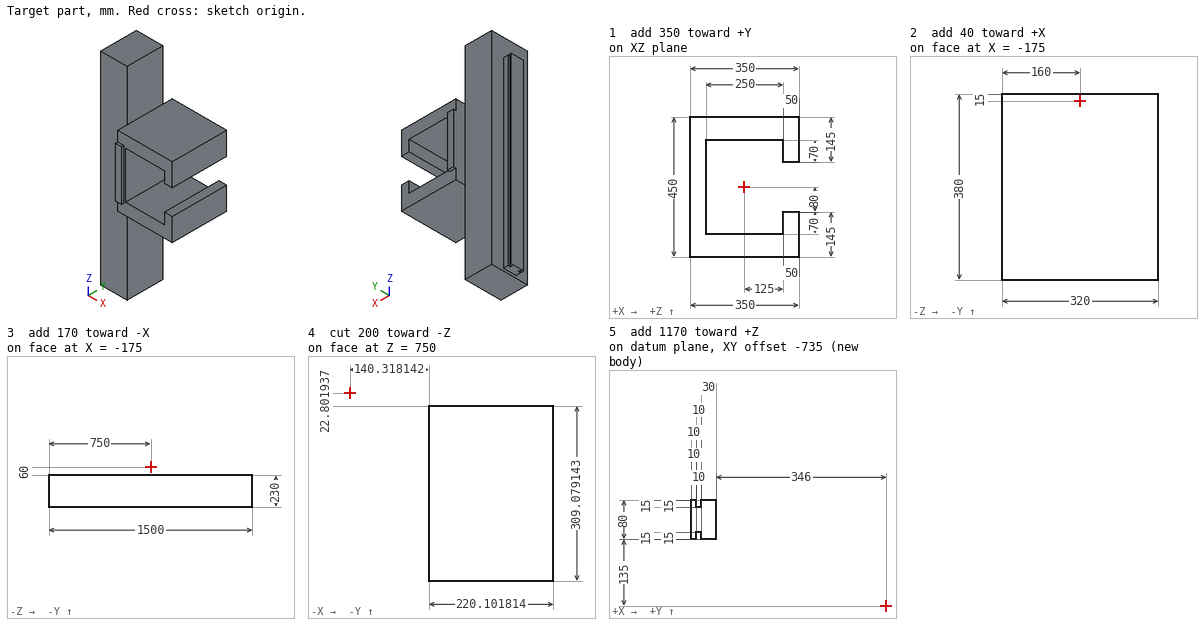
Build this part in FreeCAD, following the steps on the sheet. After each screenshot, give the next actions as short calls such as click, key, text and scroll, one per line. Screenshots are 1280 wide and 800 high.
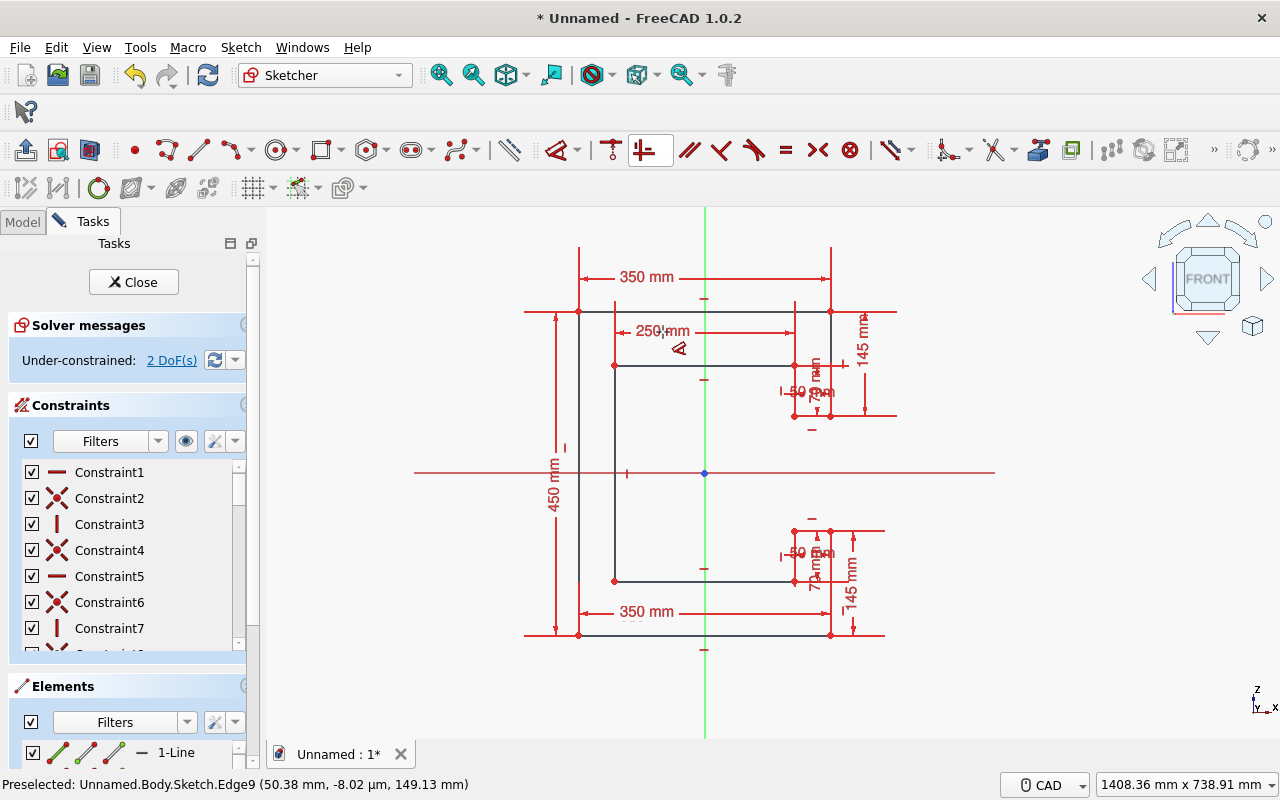
click(795, 531)
click(829, 502)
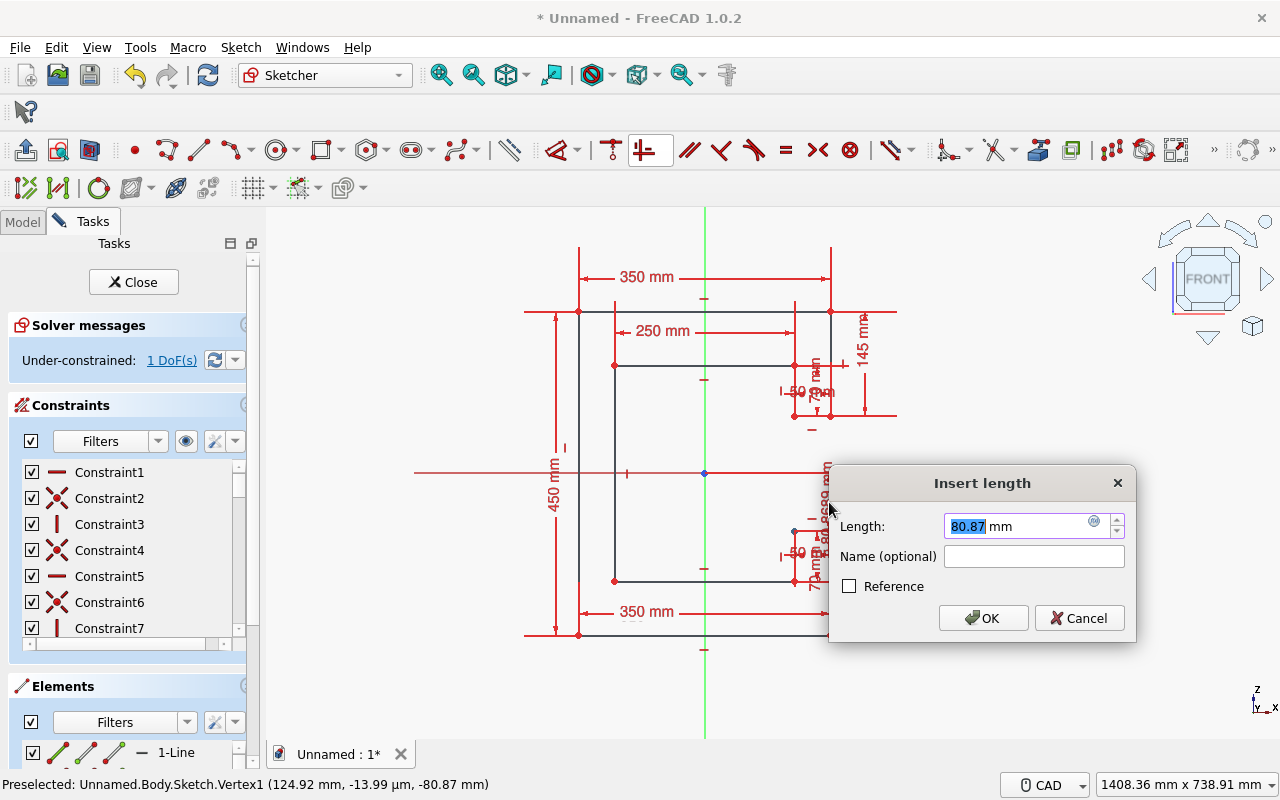
text(80)
key(Return)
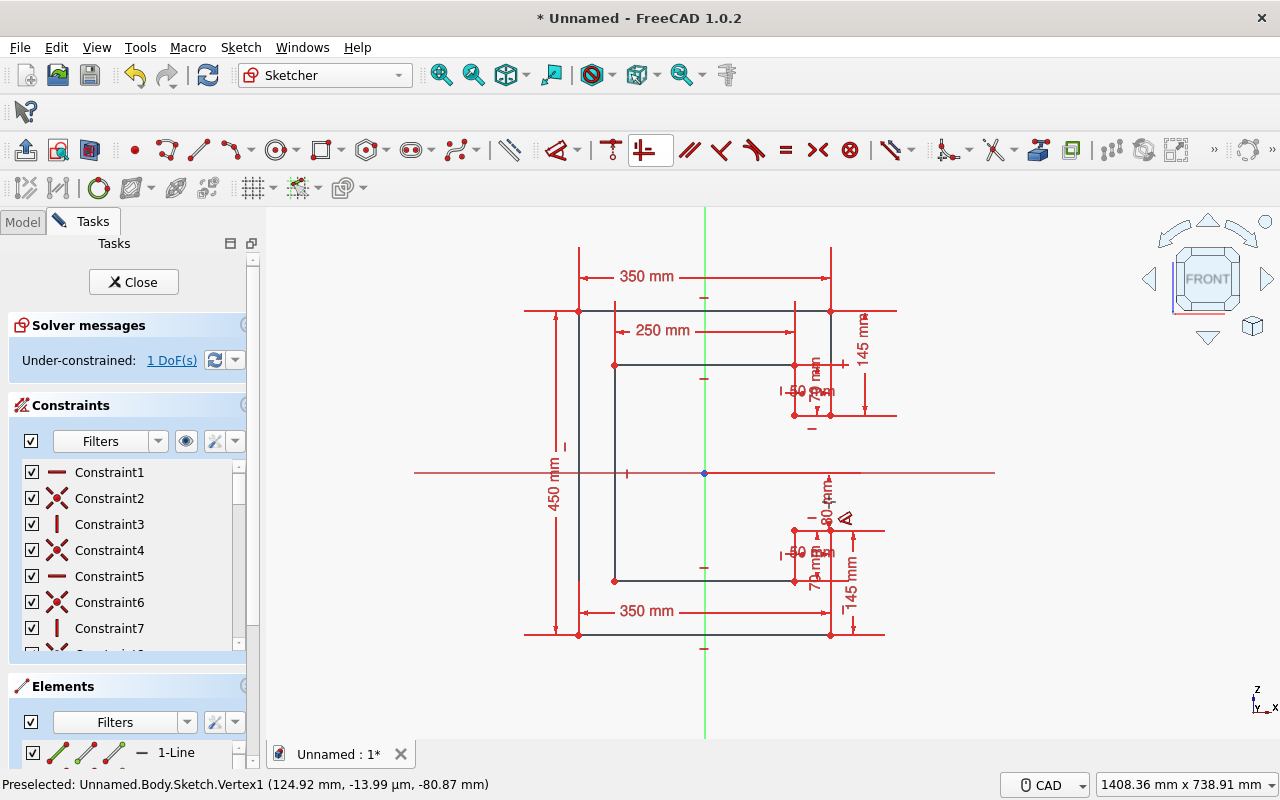
click(795, 531)
click(729, 565)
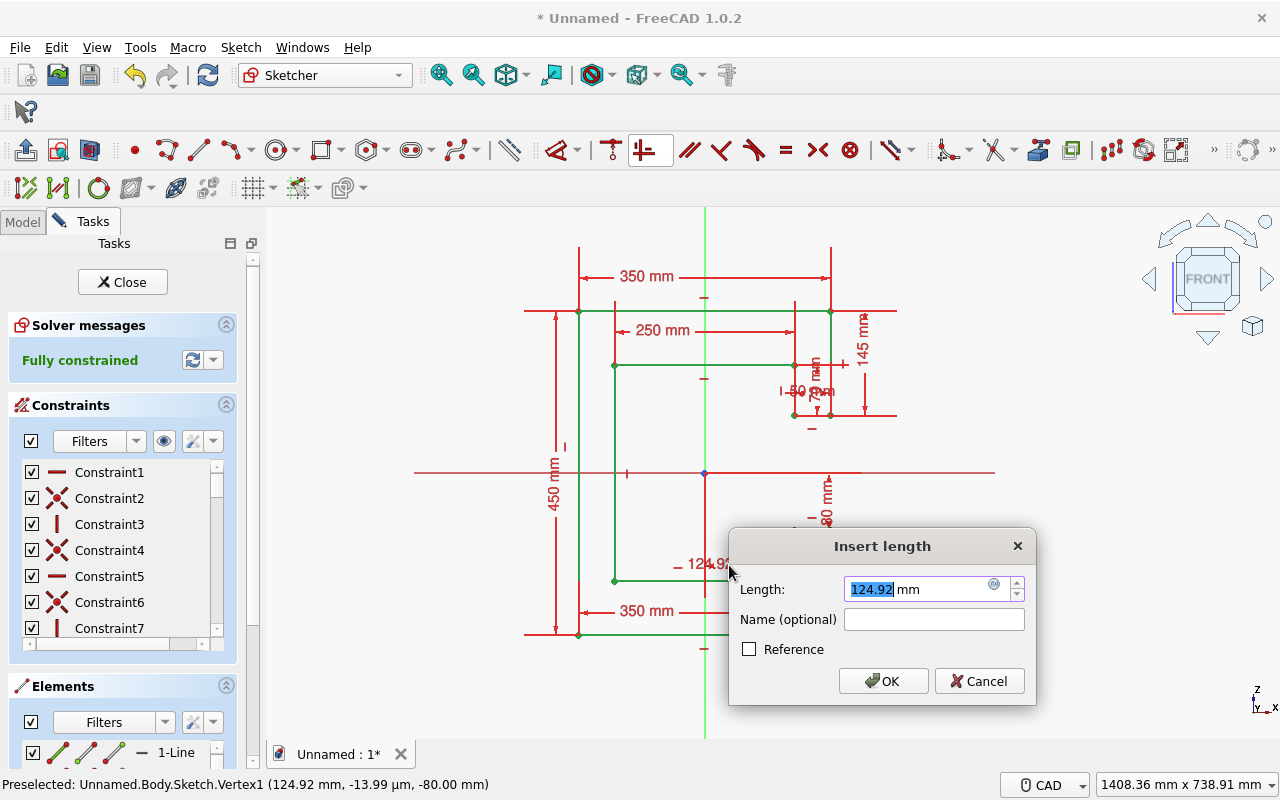
text(125)
key(Return)
key(Escape)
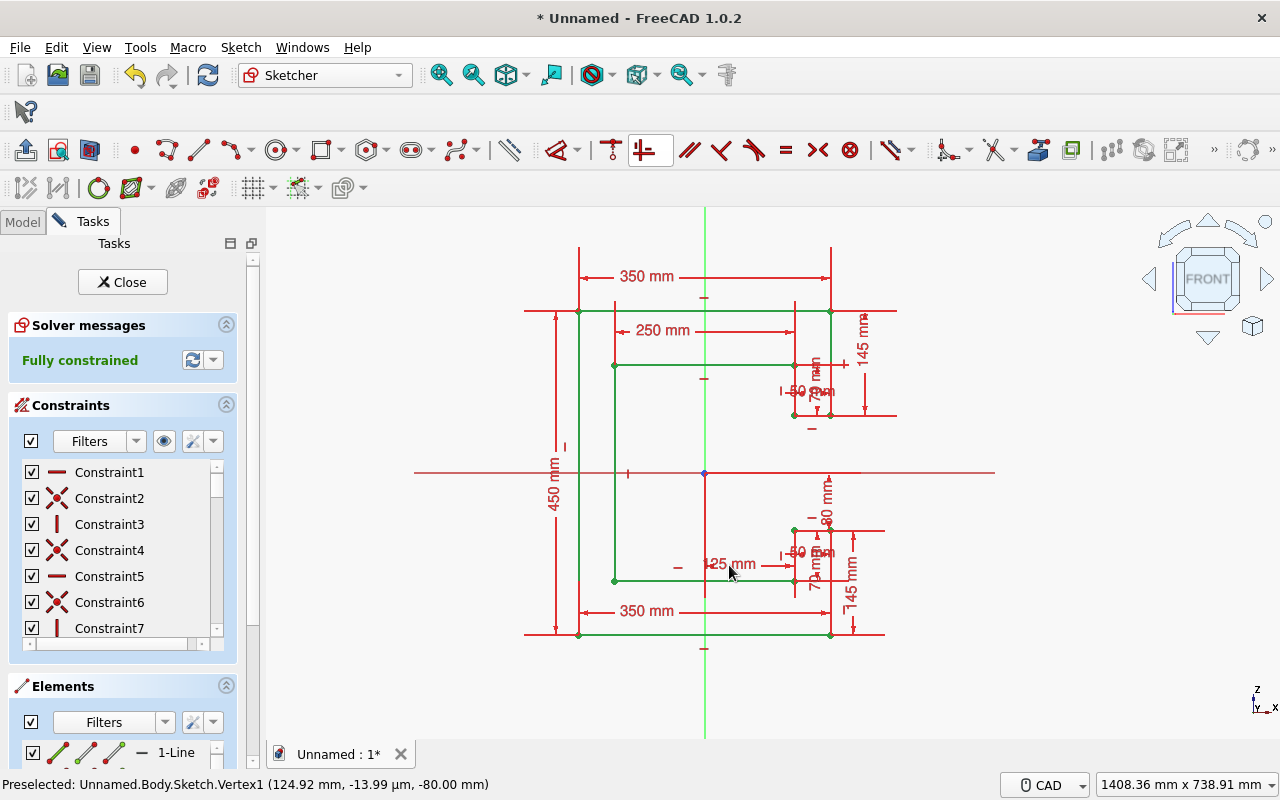
click(123, 282)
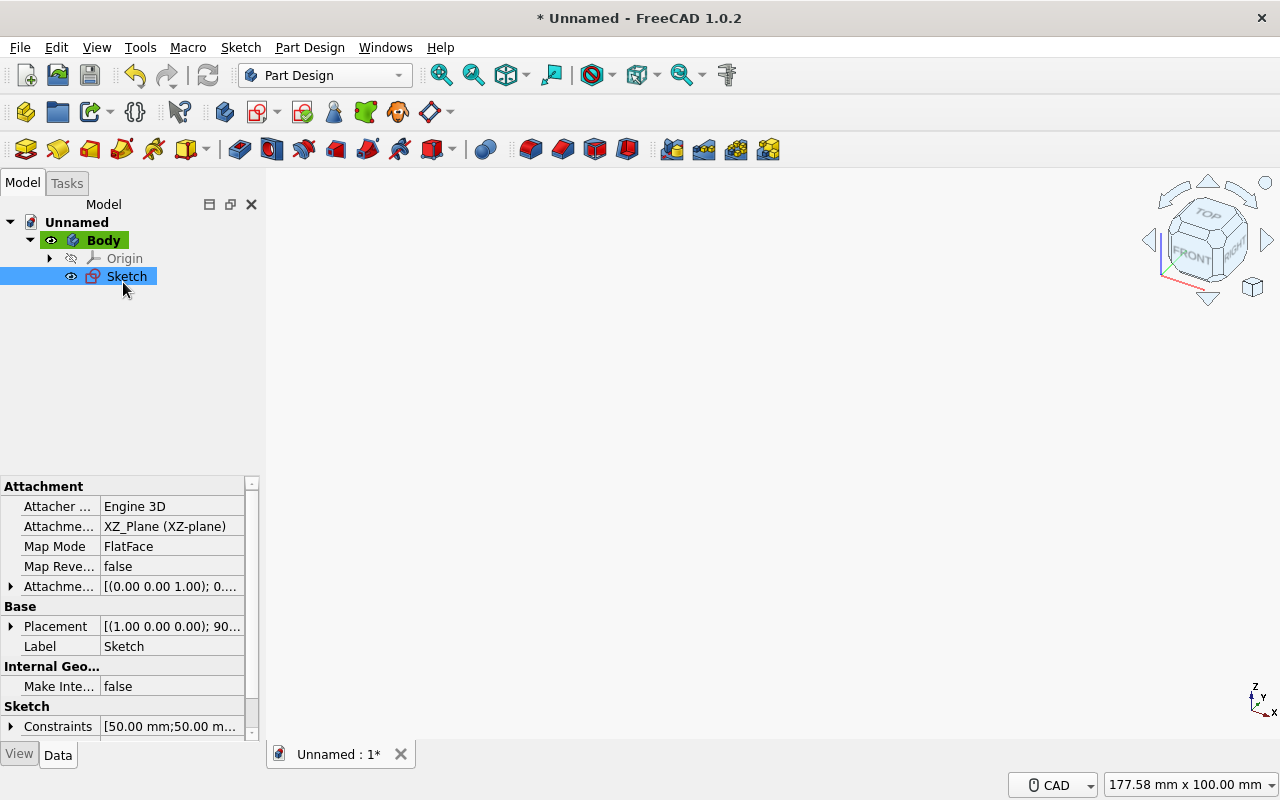
click(26, 150)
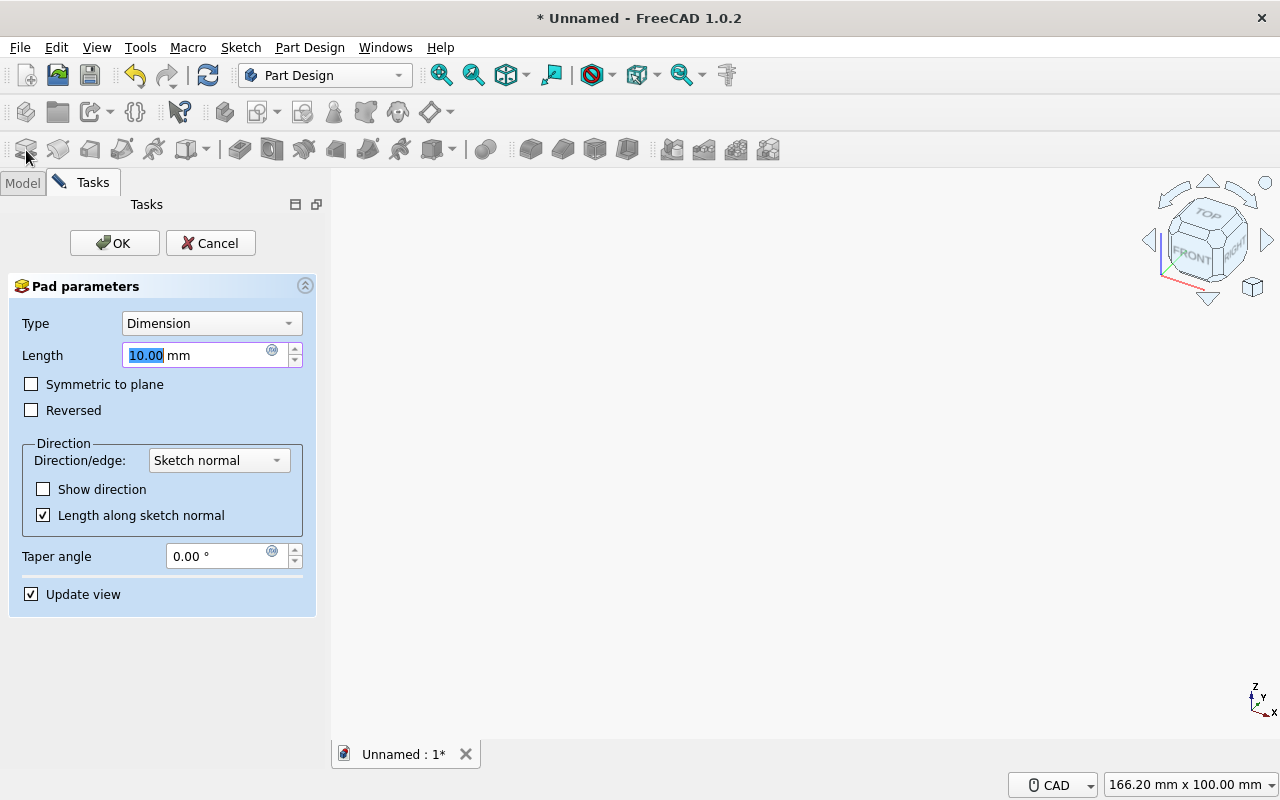
text(350)
key(Tab)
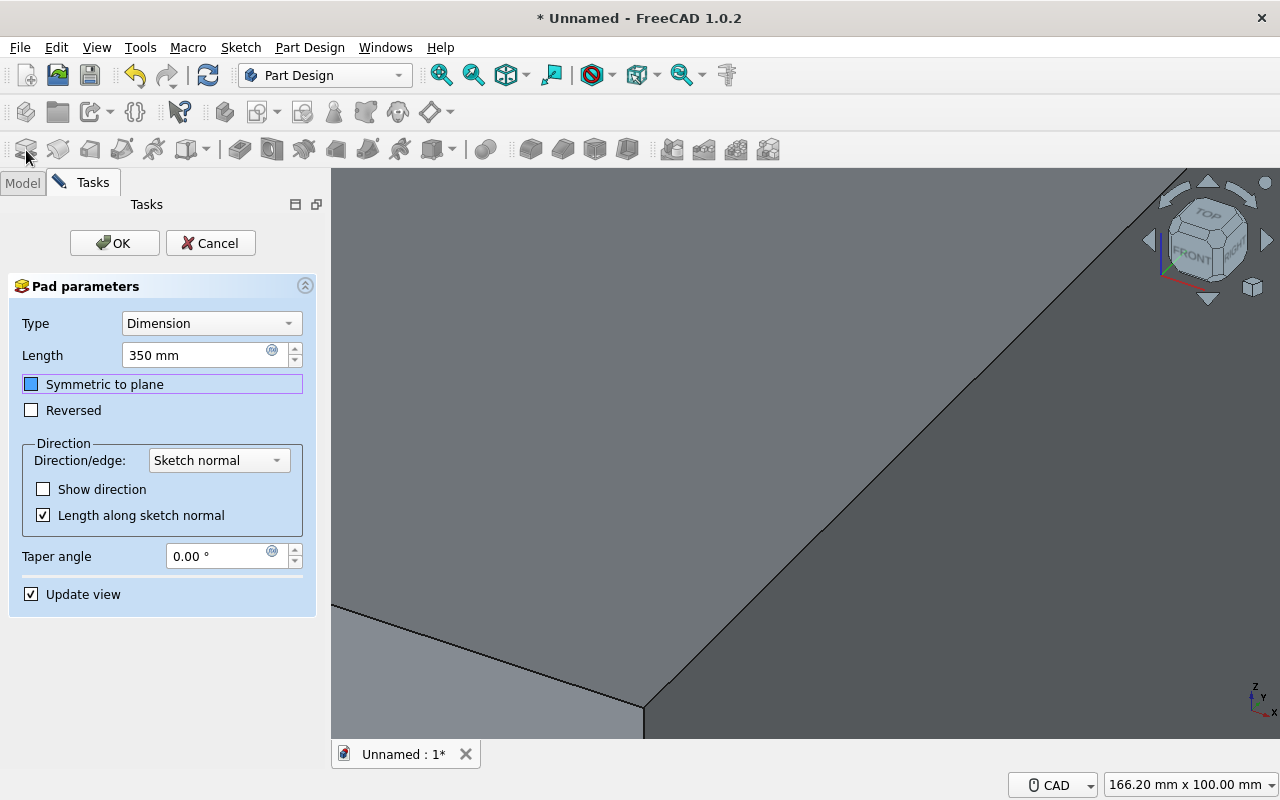
click(30, 410)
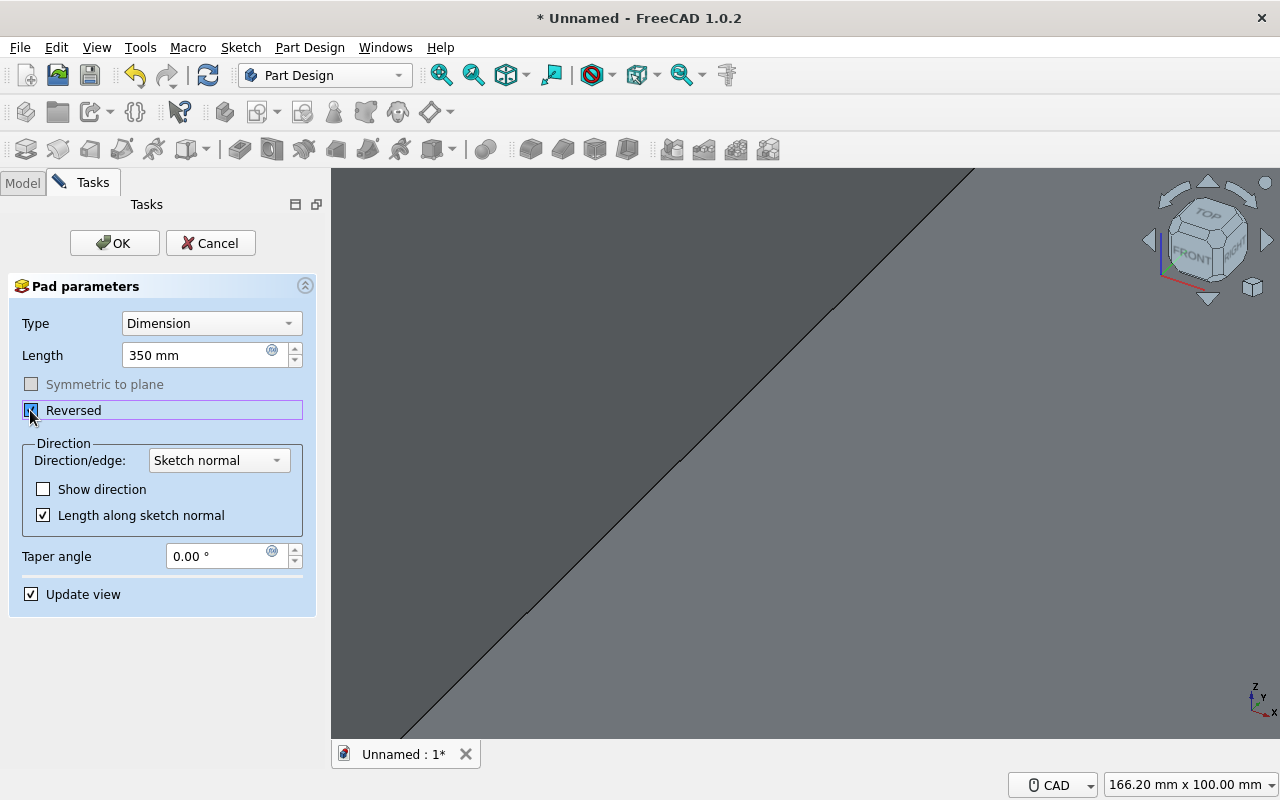
click(115, 243)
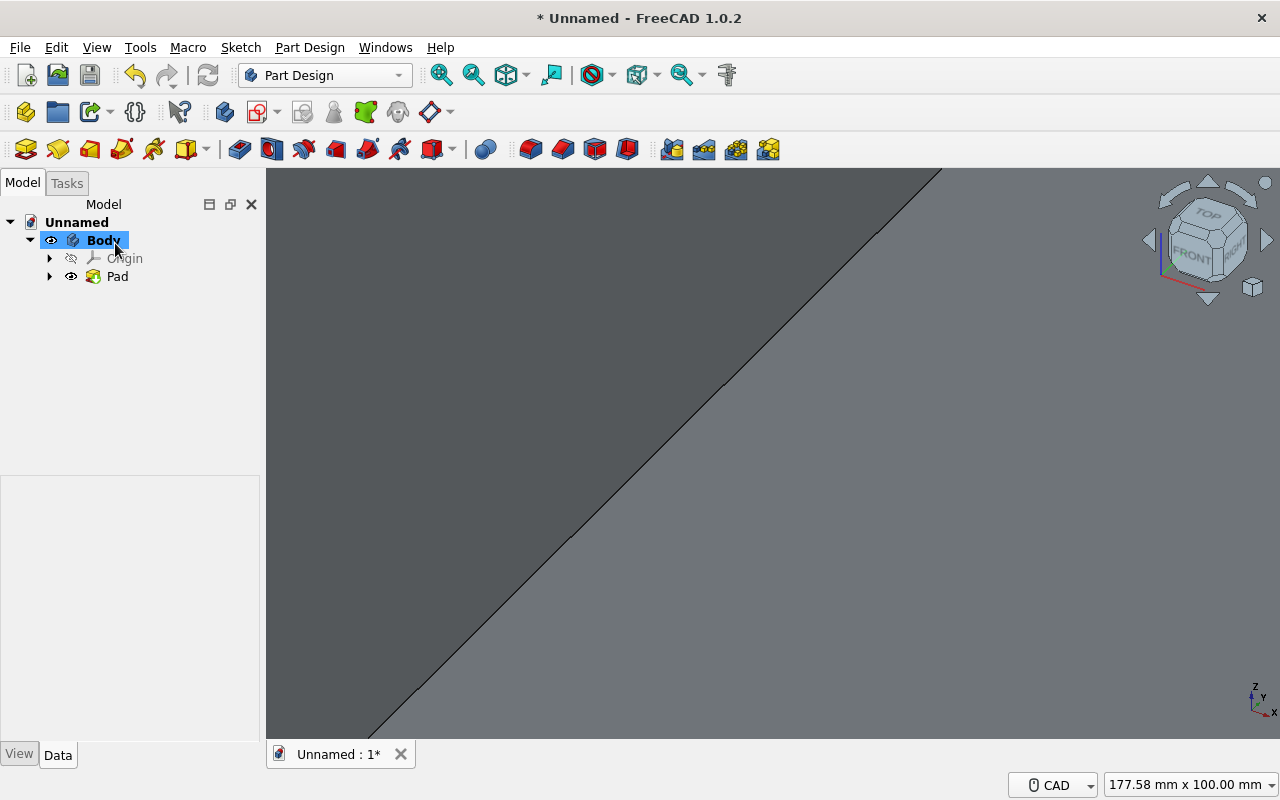
click(442, 76)